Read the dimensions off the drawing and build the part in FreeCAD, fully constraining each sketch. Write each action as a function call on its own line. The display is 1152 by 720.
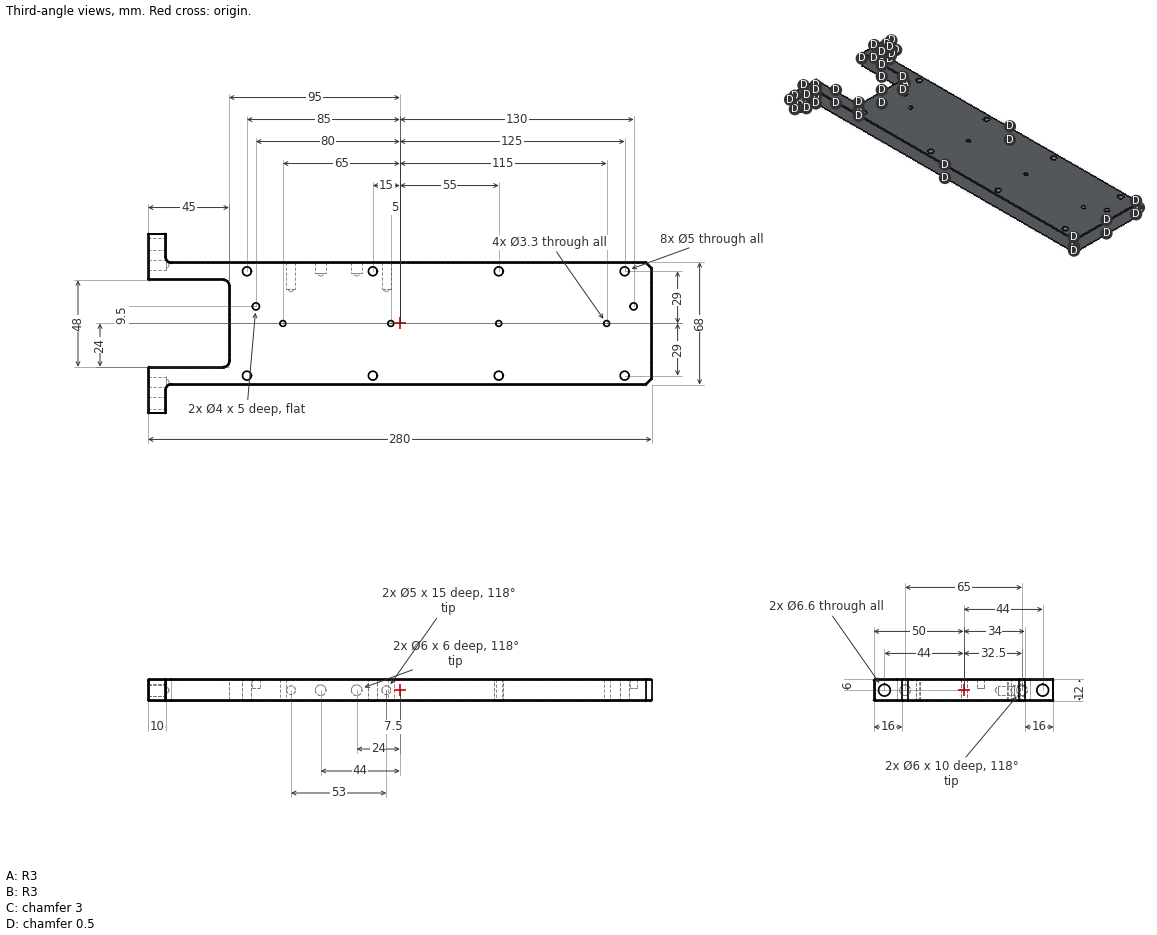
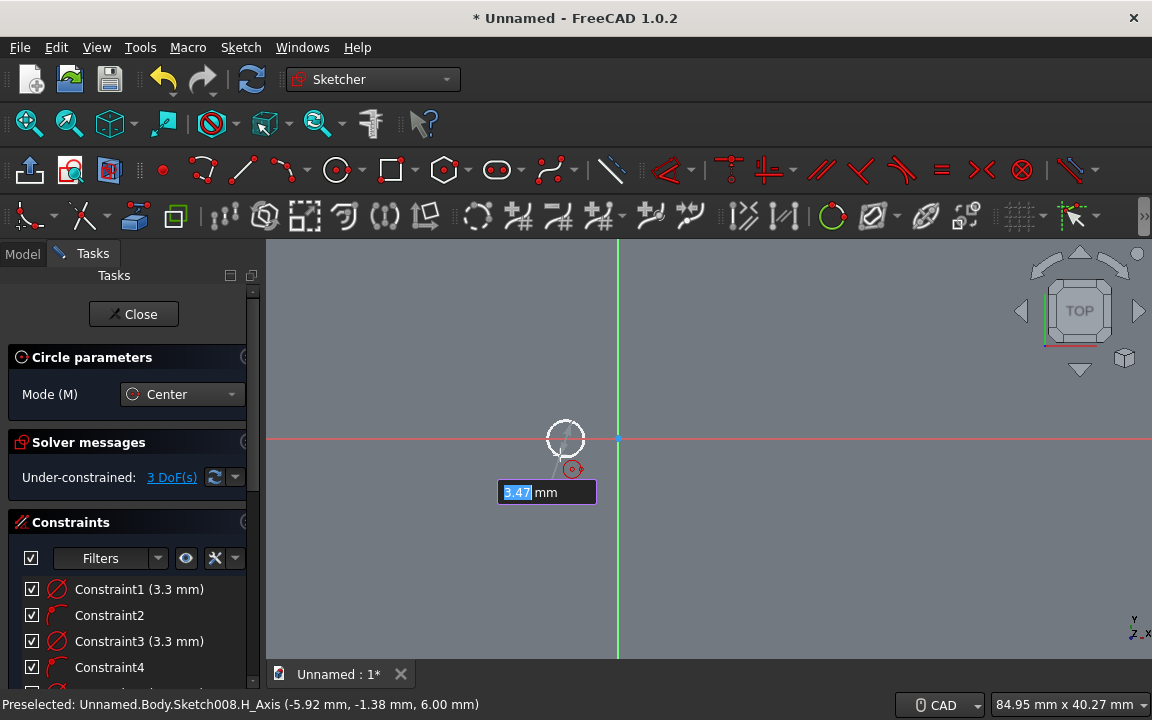
text(3.3)
key(Return)
key(Escape)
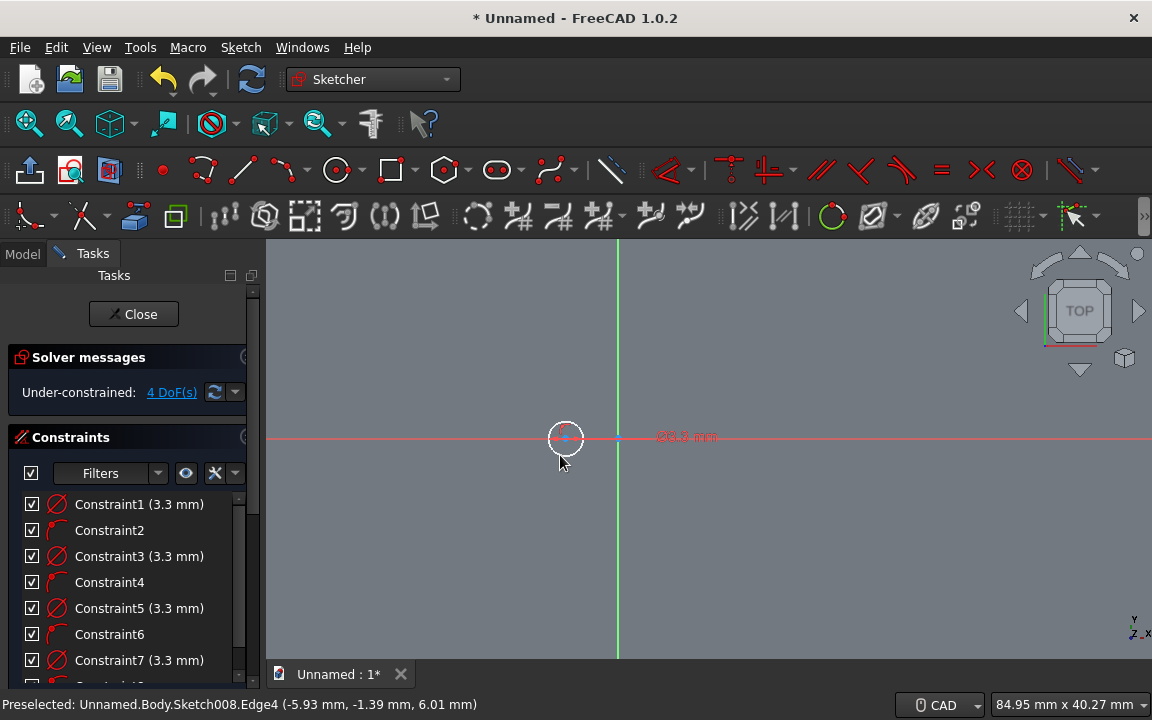
key(d)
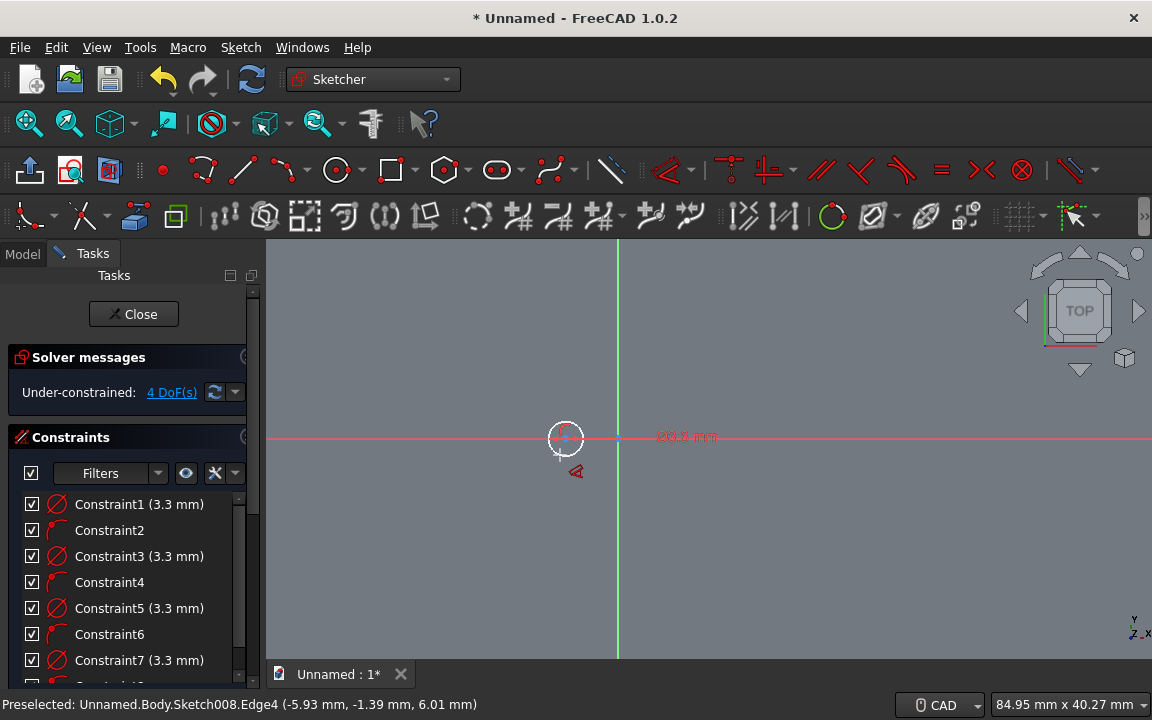
click(566, 439)
click(592, 473)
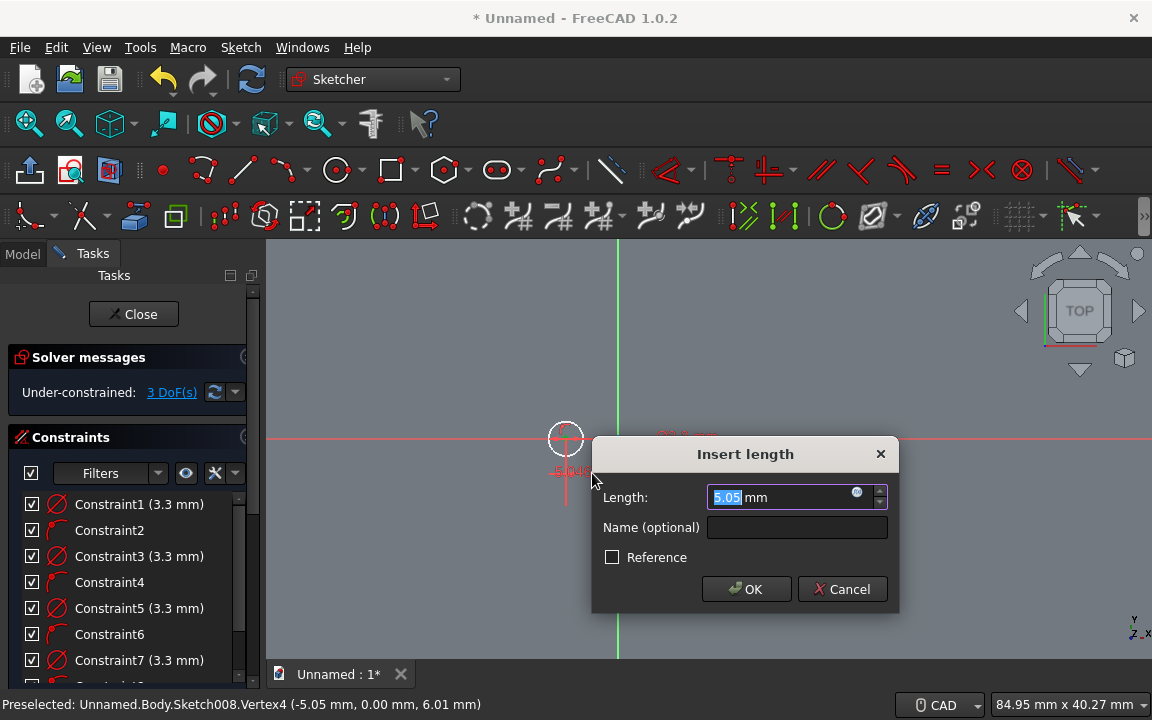
text(5)
key(Return)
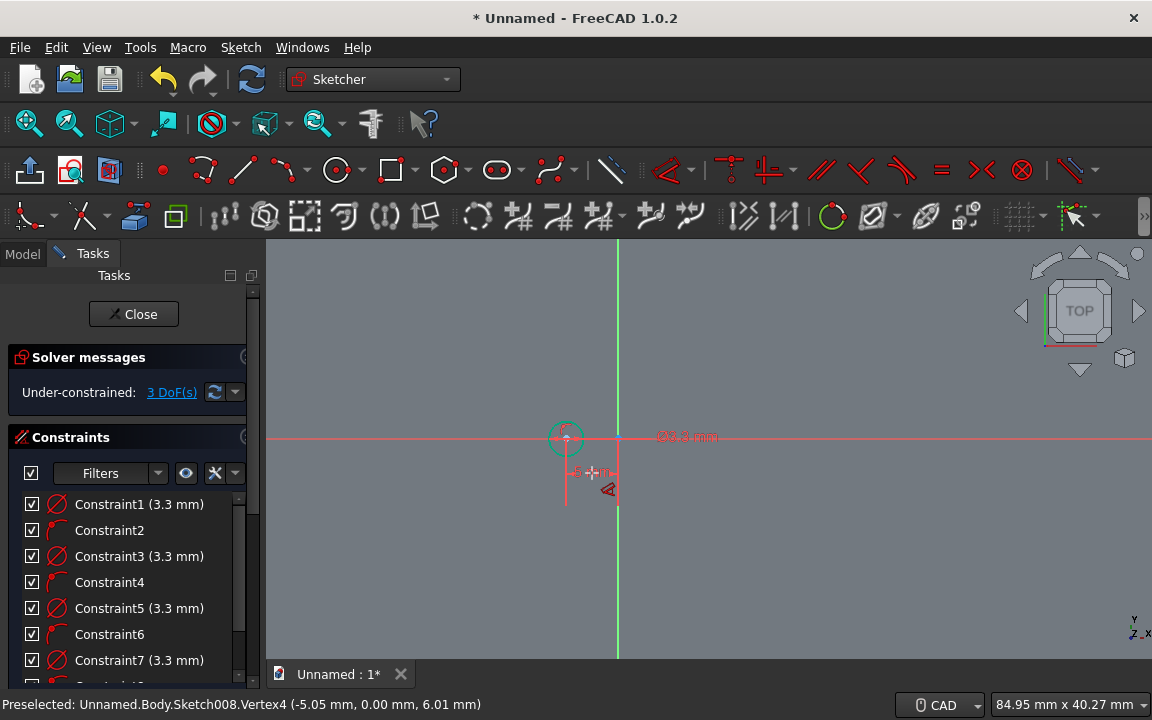
scroll(562, 452, down, 7)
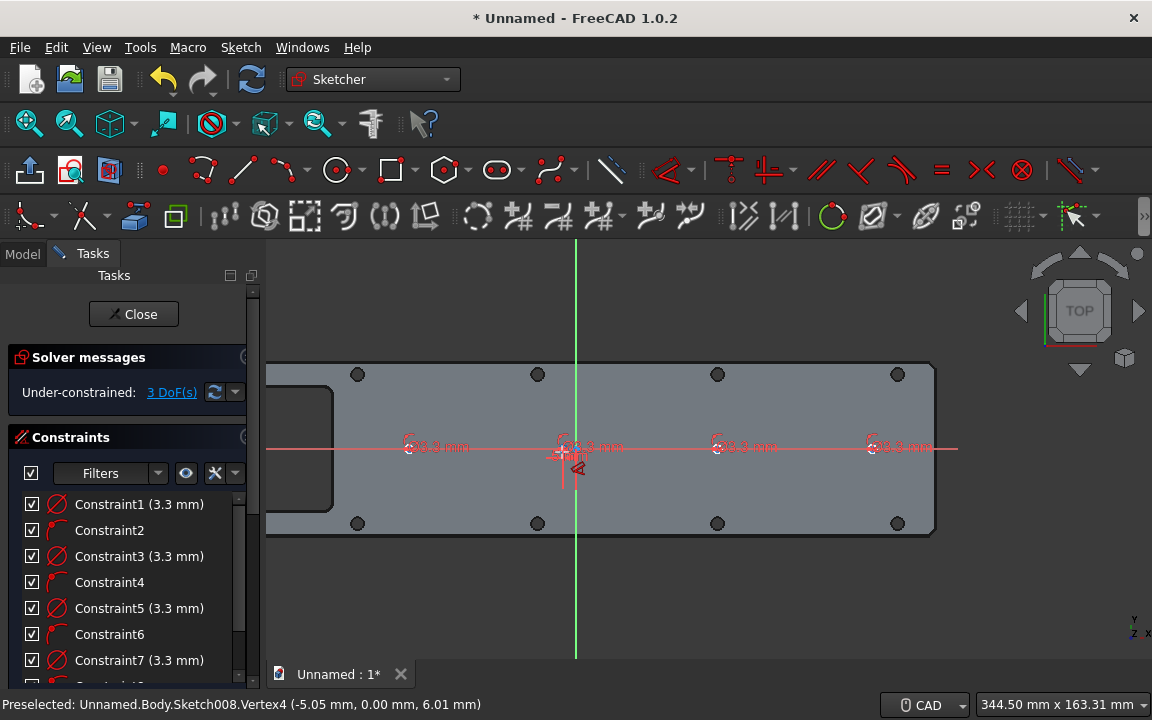
click(717, 449)
click(647, 483)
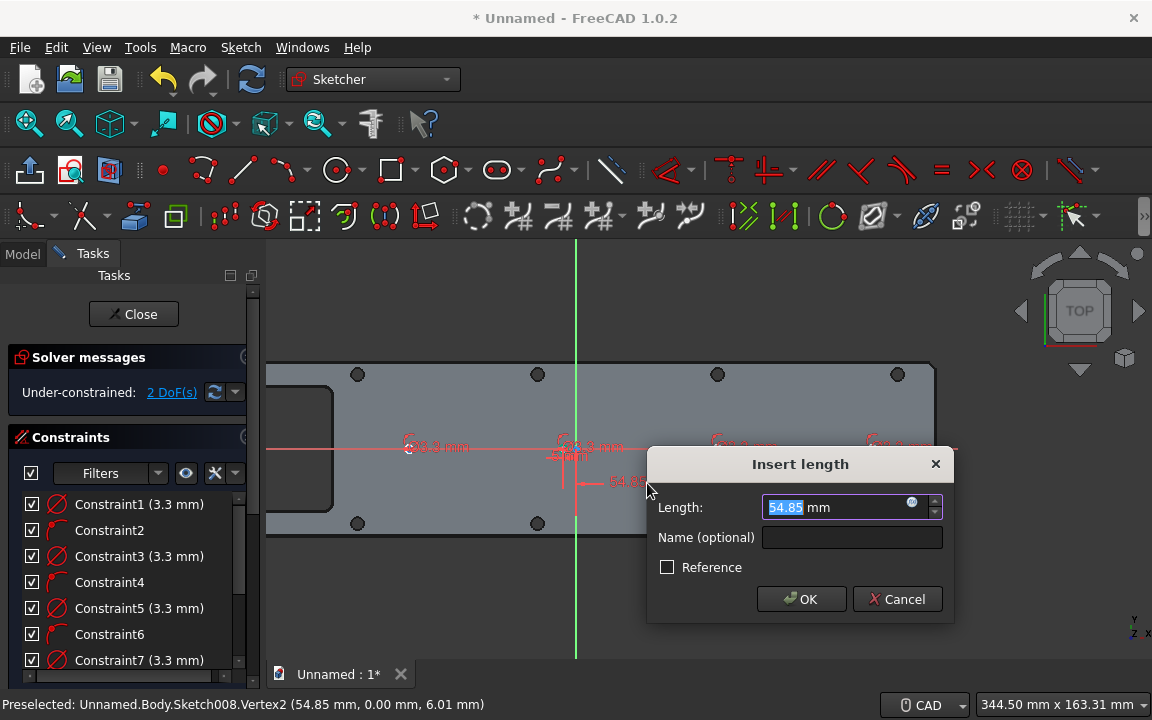
text(55)
key(Return)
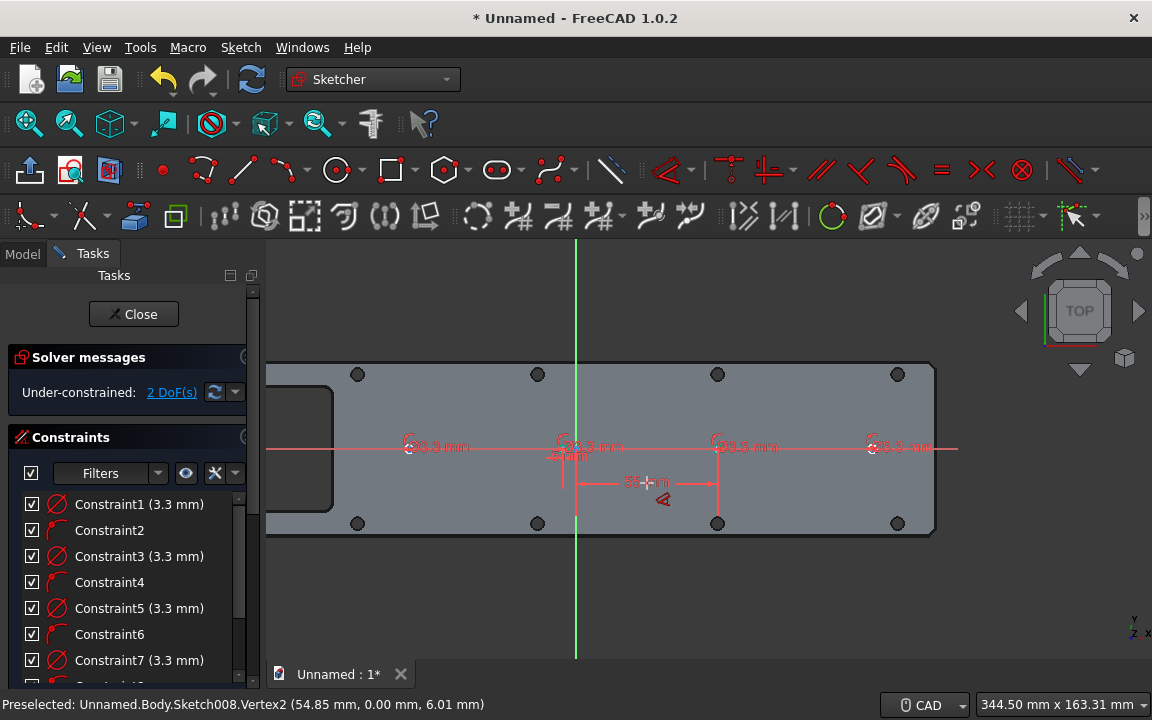
click(409, 449)
click(493, 483)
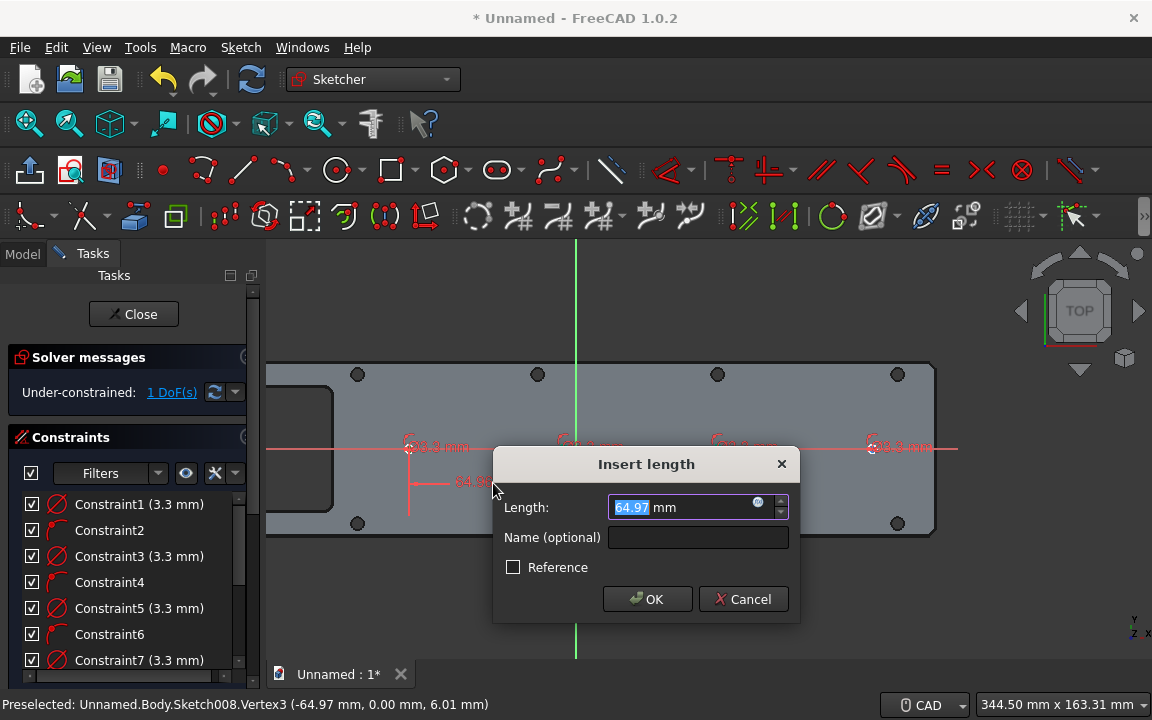
text(65)
key(Return)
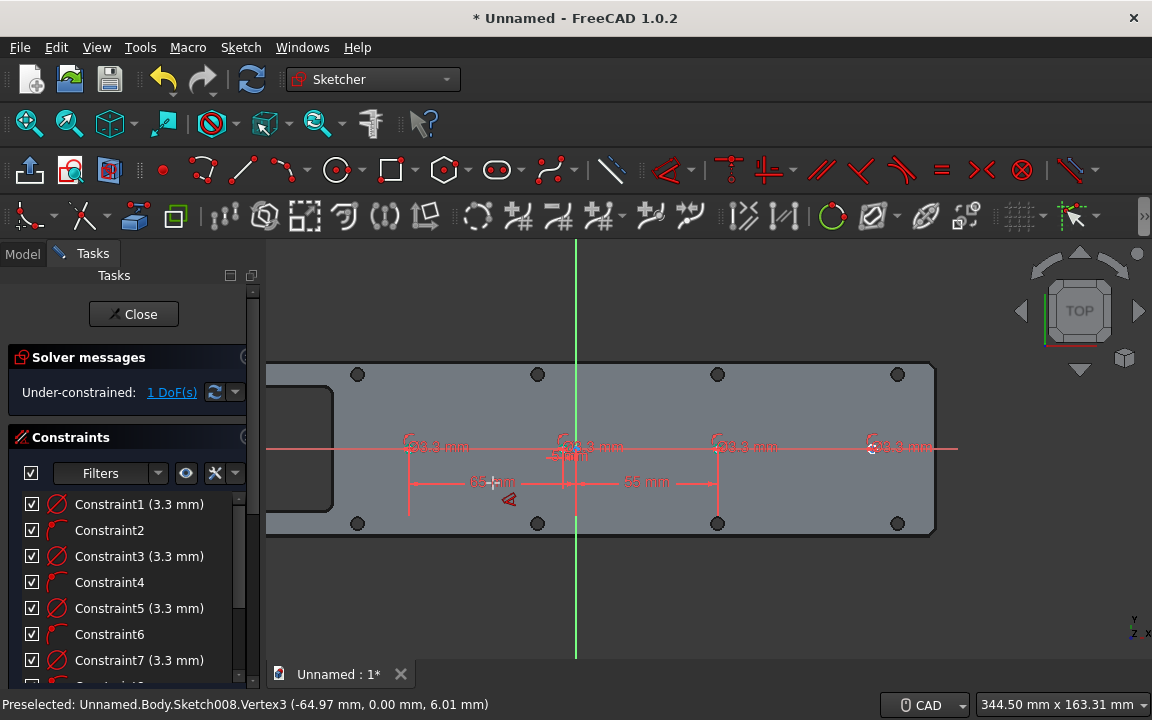
click(872, 449)
click(724, 483)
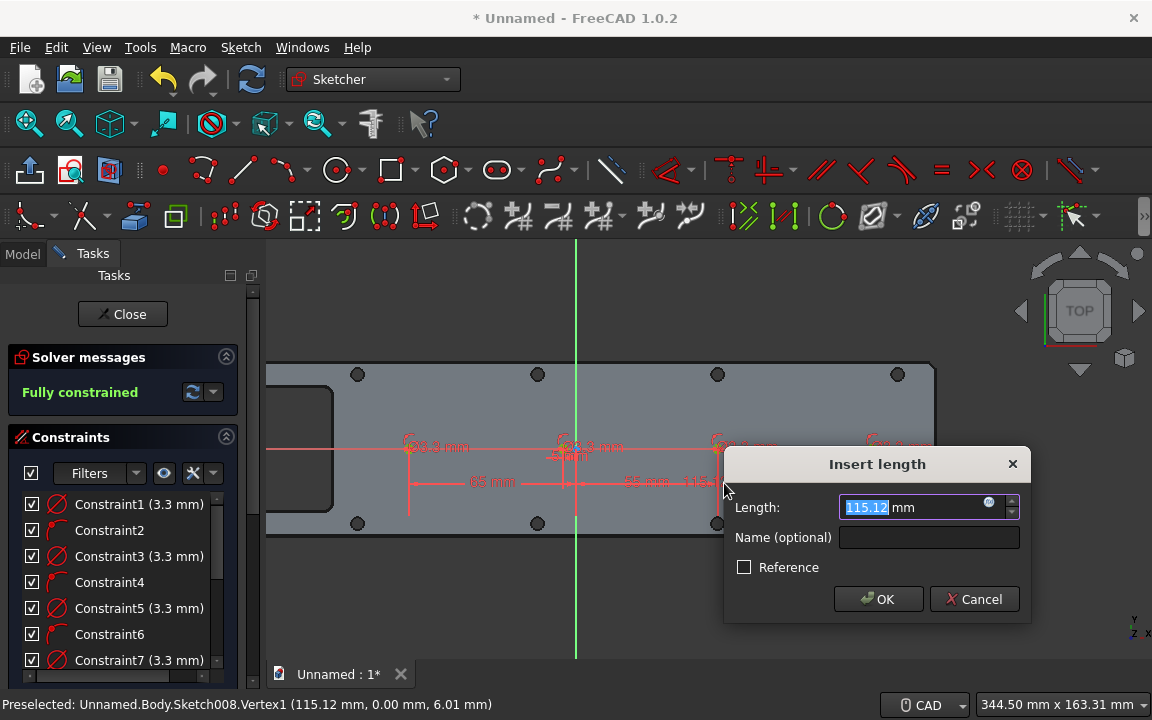
text(115)
key(Return)
key(Escape)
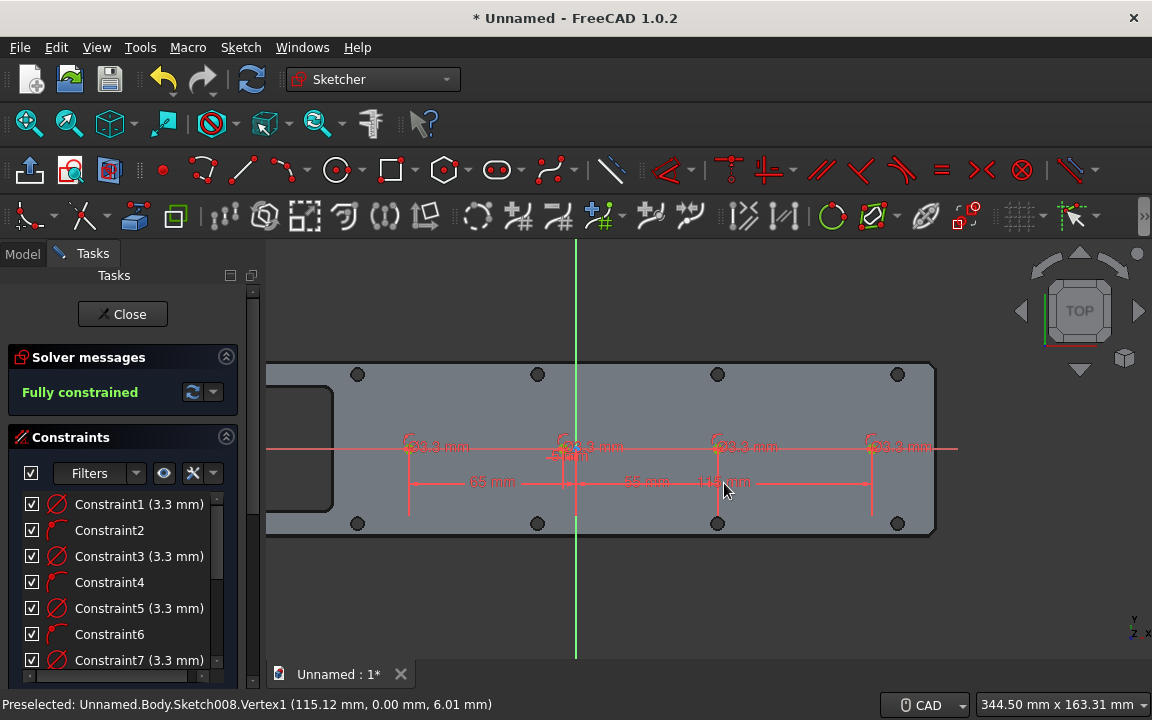
click(123, 314)